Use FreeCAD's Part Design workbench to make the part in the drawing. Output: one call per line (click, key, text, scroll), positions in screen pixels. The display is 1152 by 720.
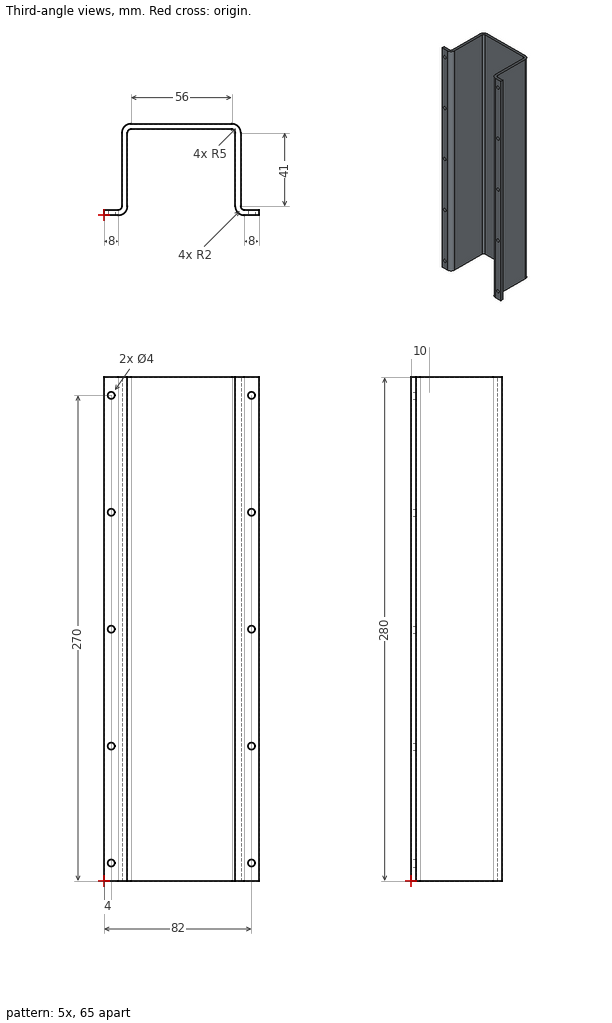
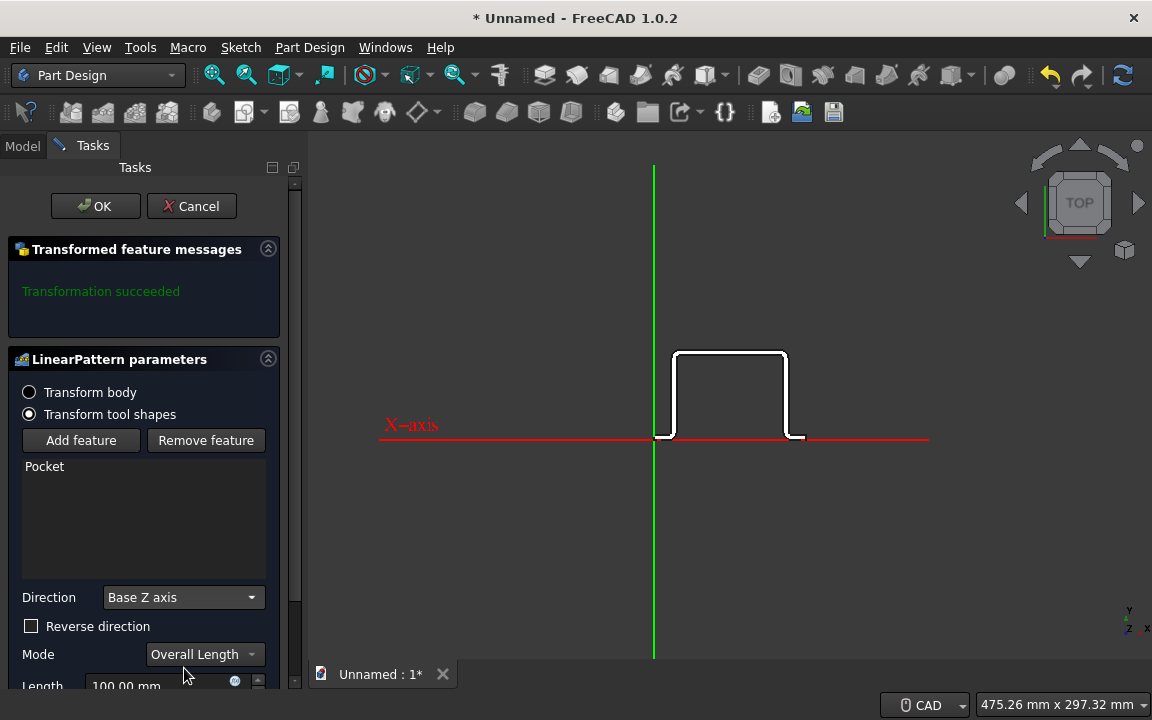
click(206, 654)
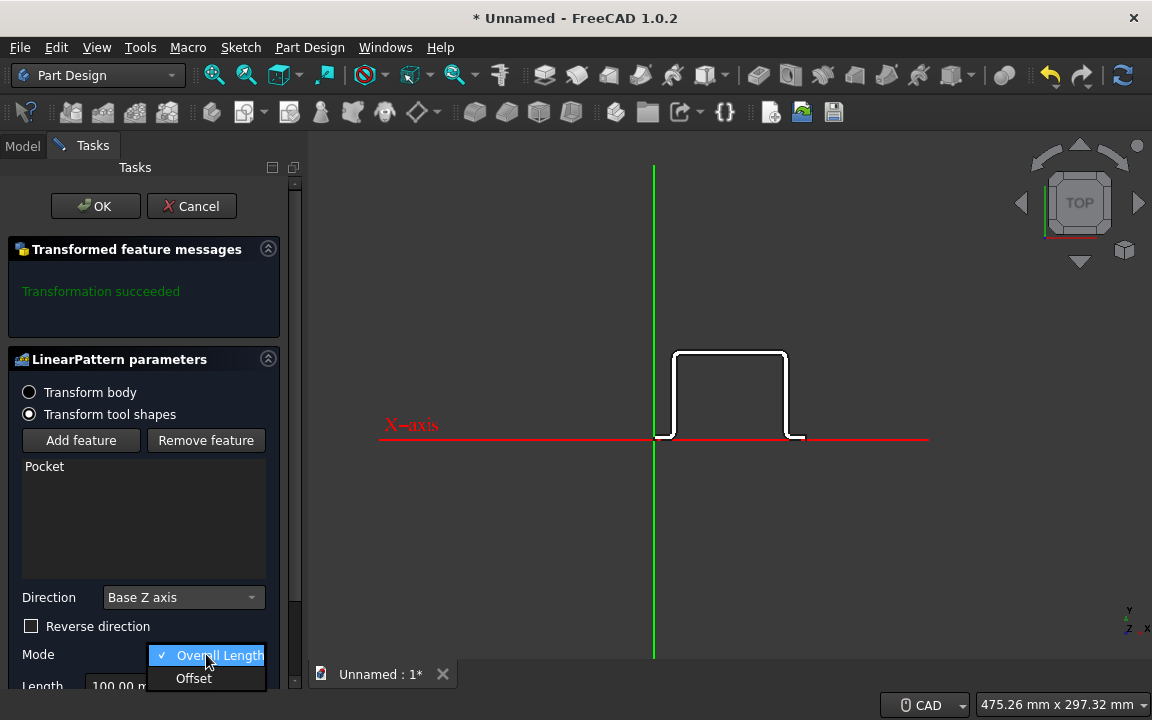
click(206, 678)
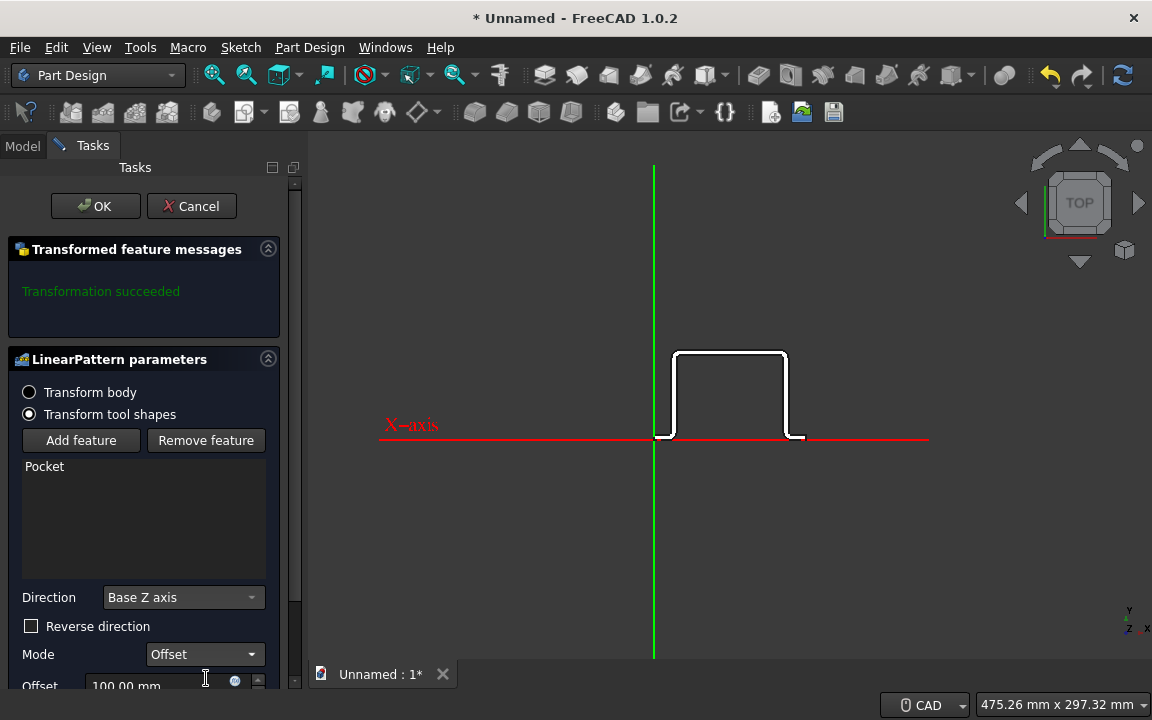
scroll(295, 432, down, 2)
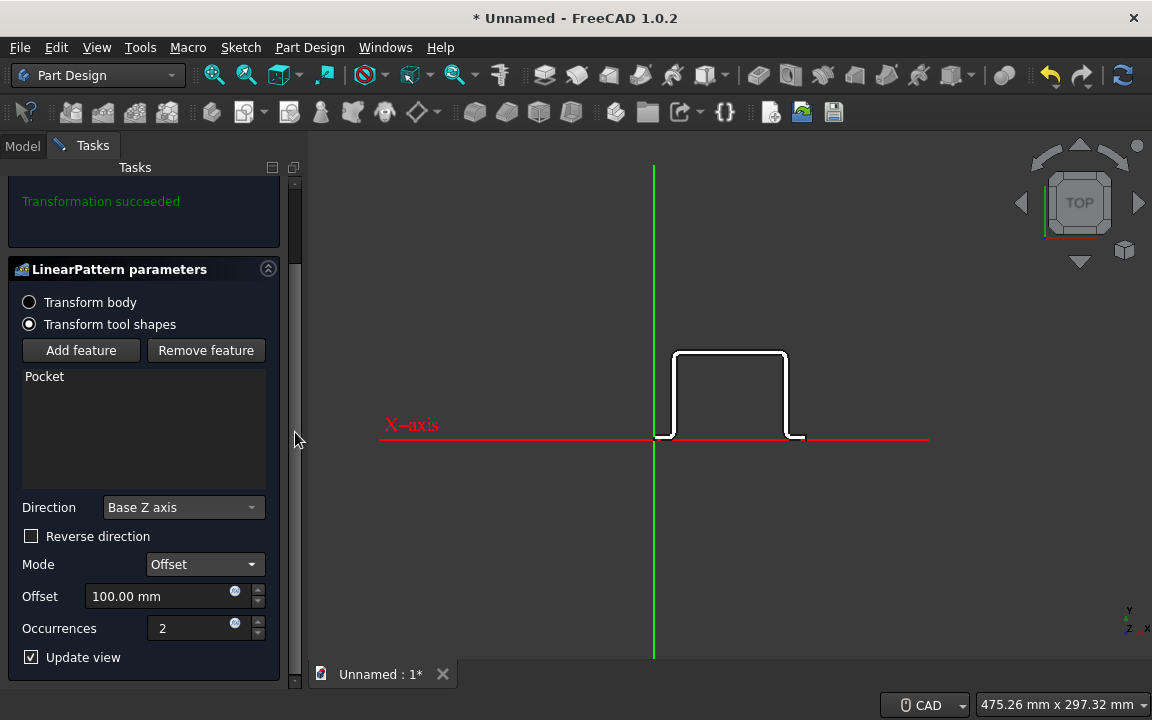
triple_click(168, 596)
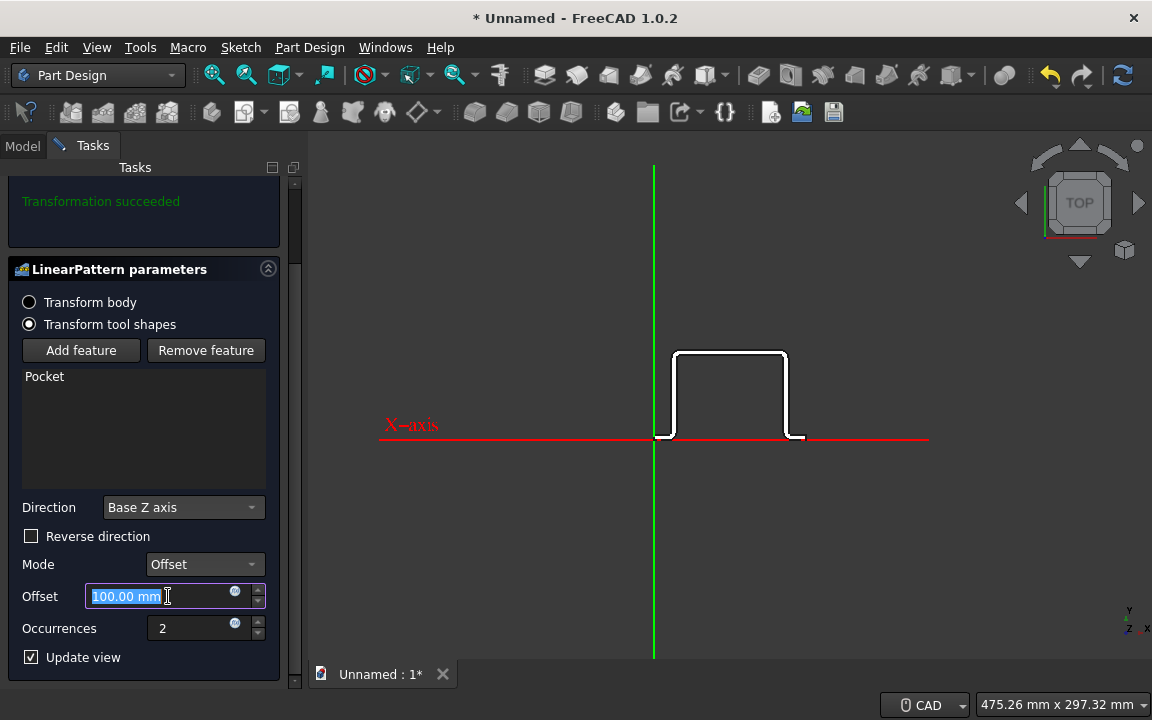
text(65)
key(Tab)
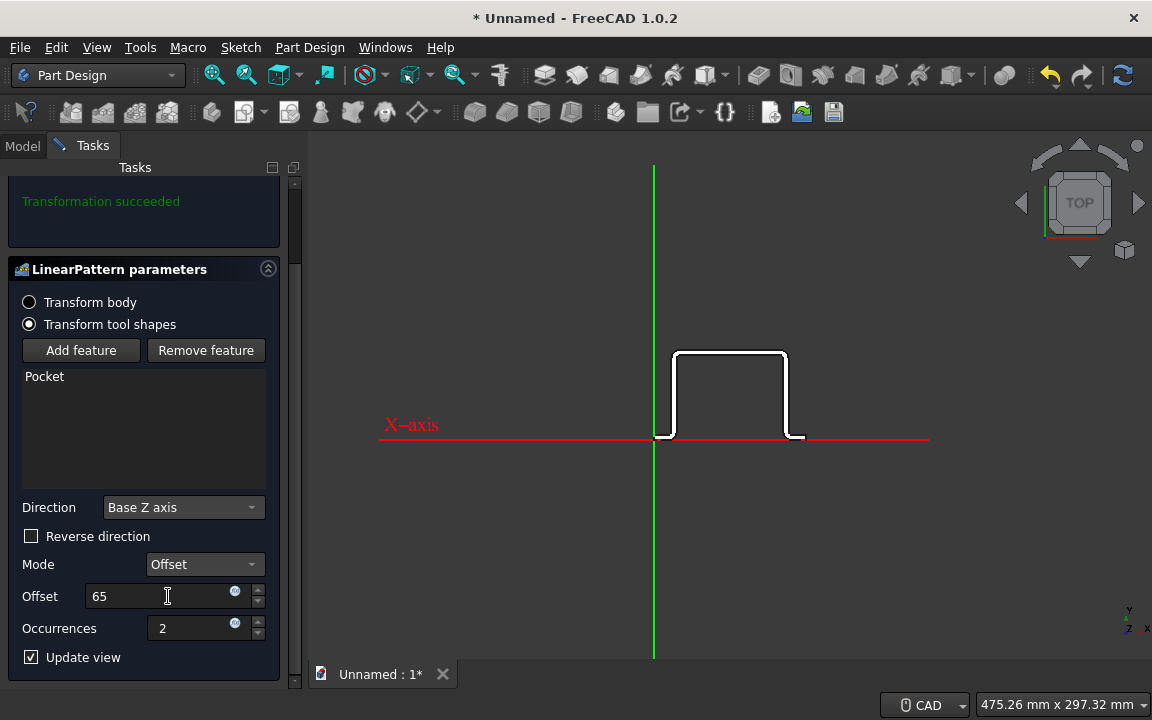
triple_click(198, 628)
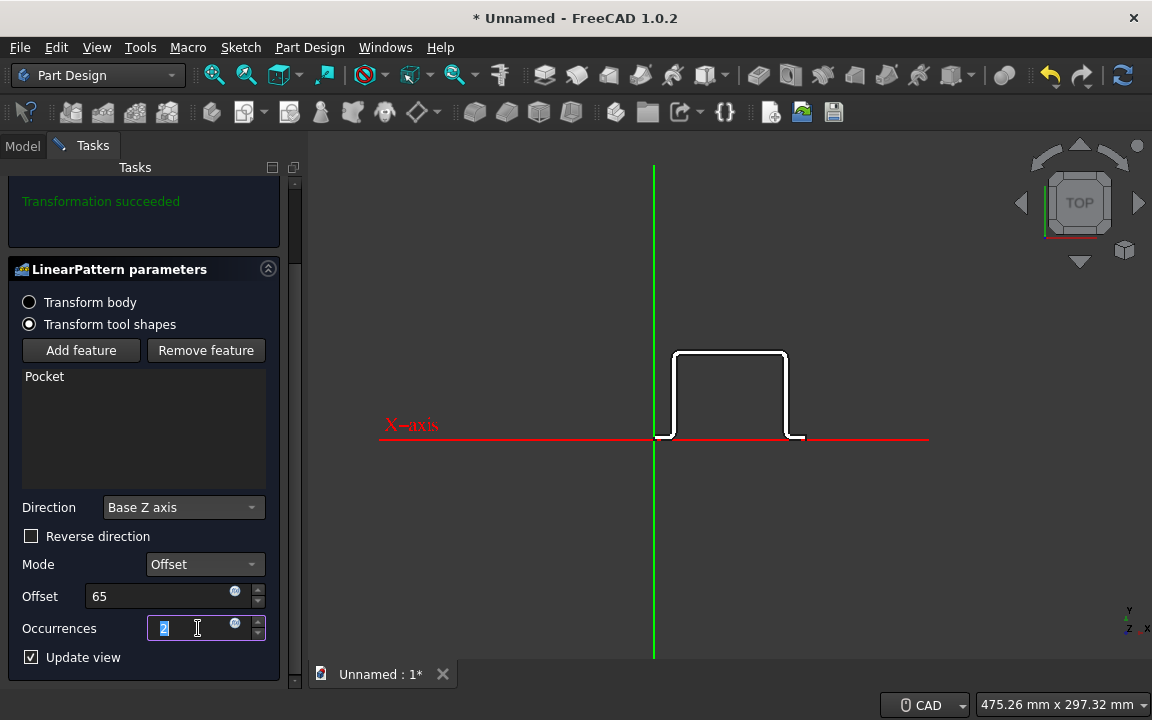
text(5)
key(Tab)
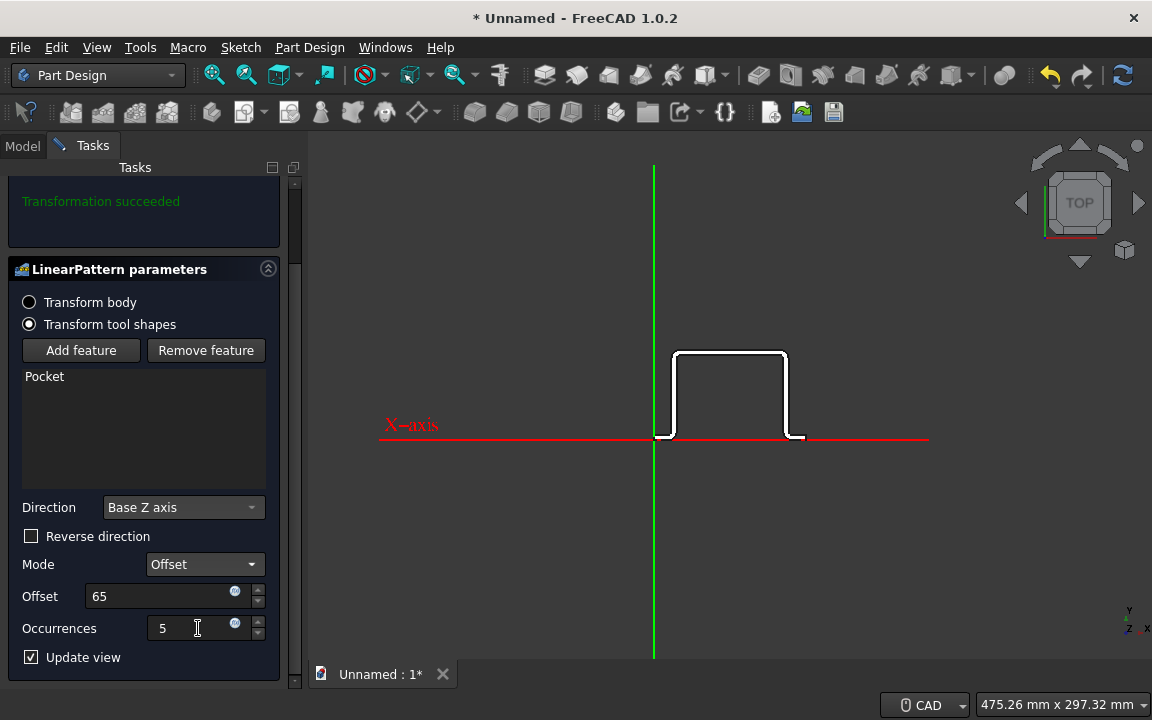
click(30, 536)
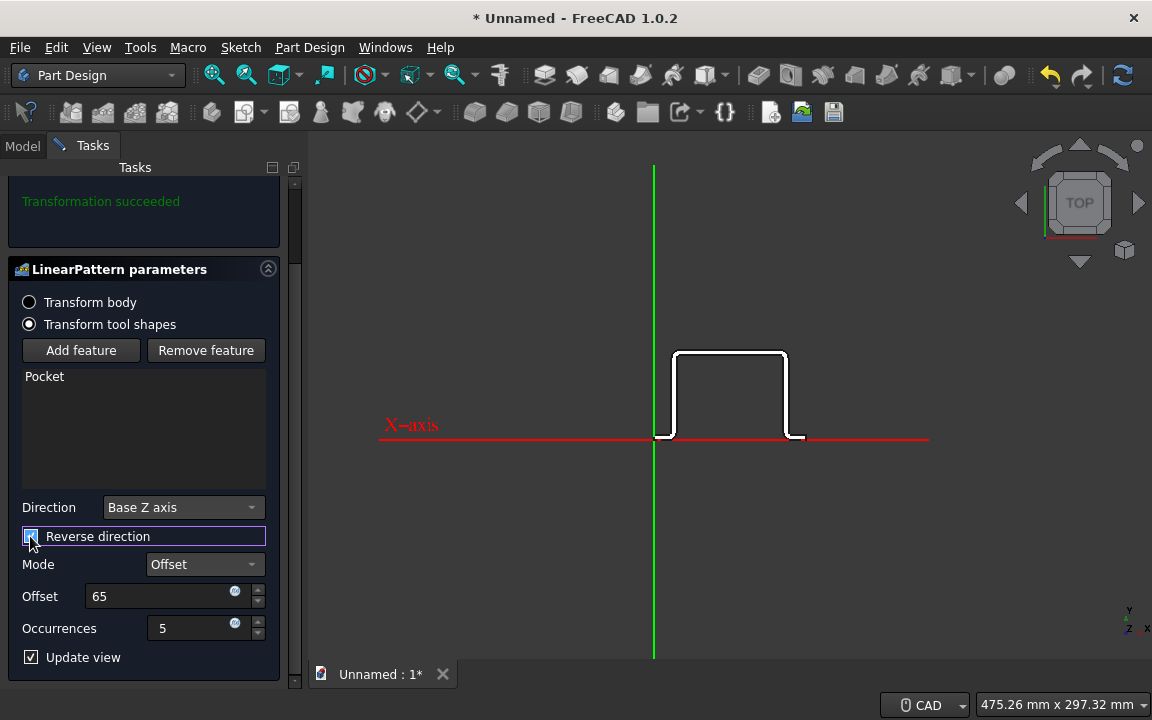
scroll(295, 432, up, 3)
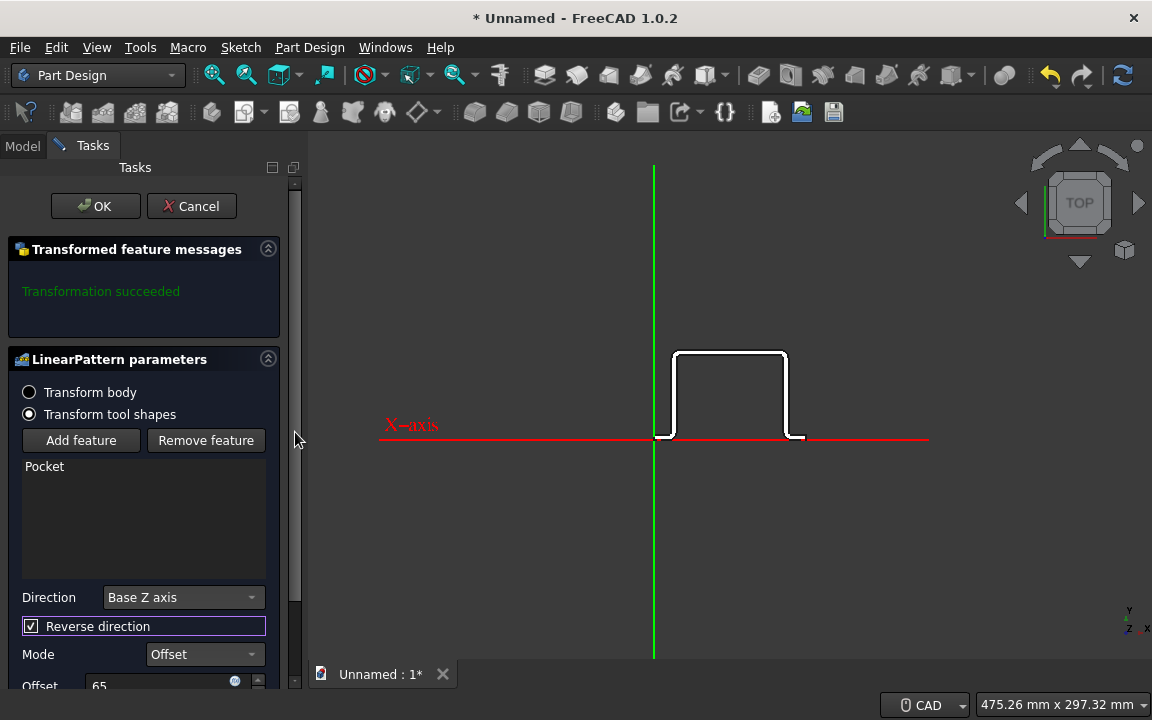
click(96, 206)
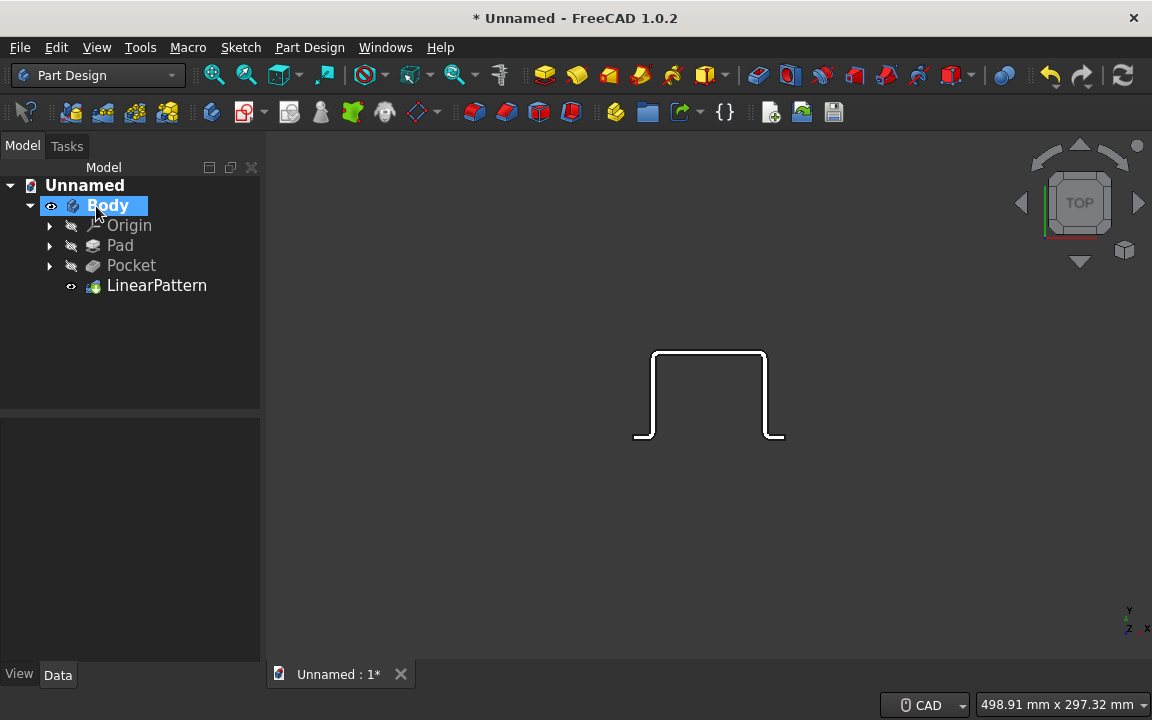
key(0)